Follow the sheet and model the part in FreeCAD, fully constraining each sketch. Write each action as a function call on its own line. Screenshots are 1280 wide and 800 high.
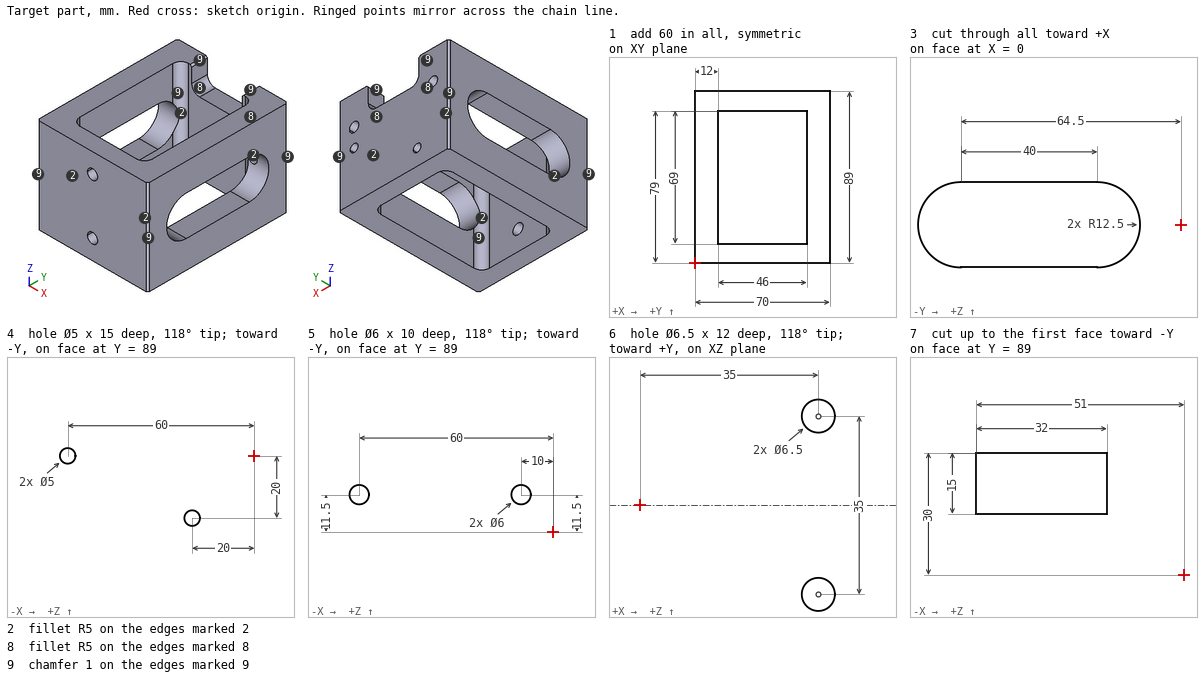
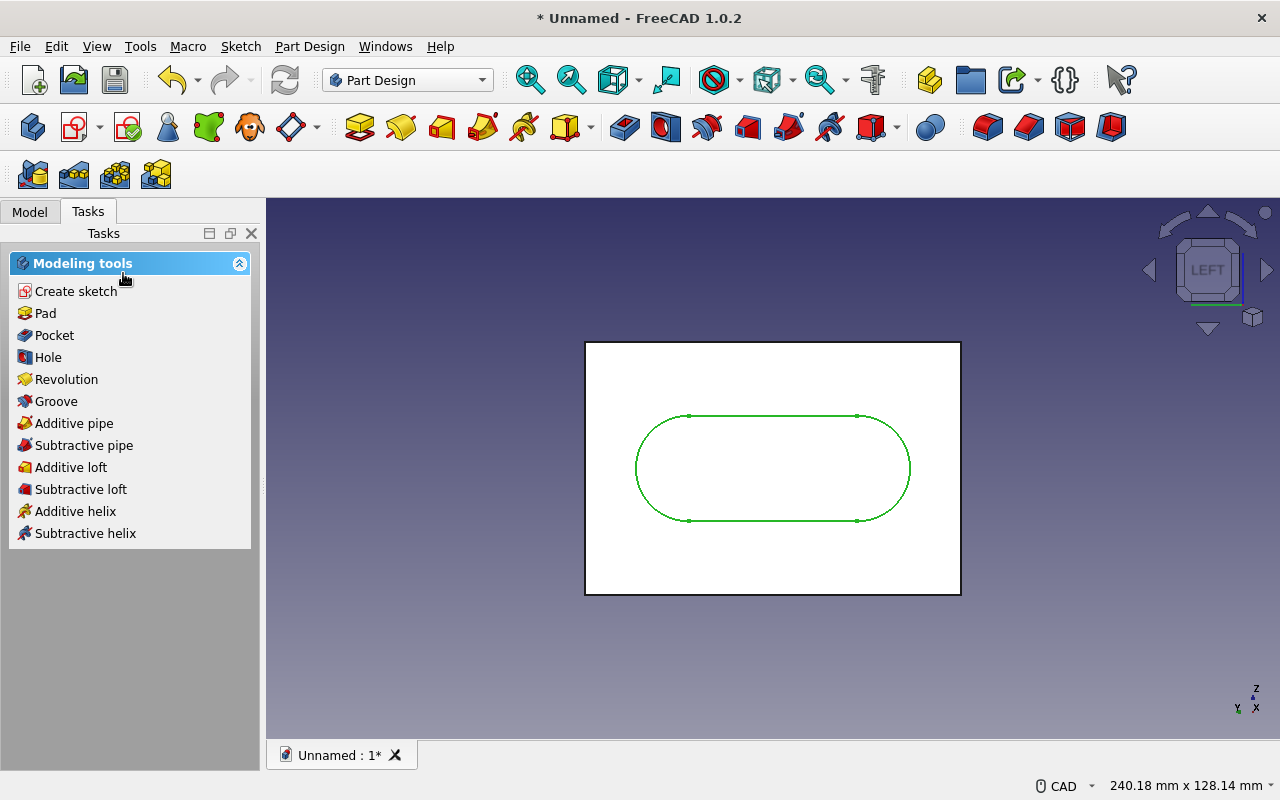
click(625, 128)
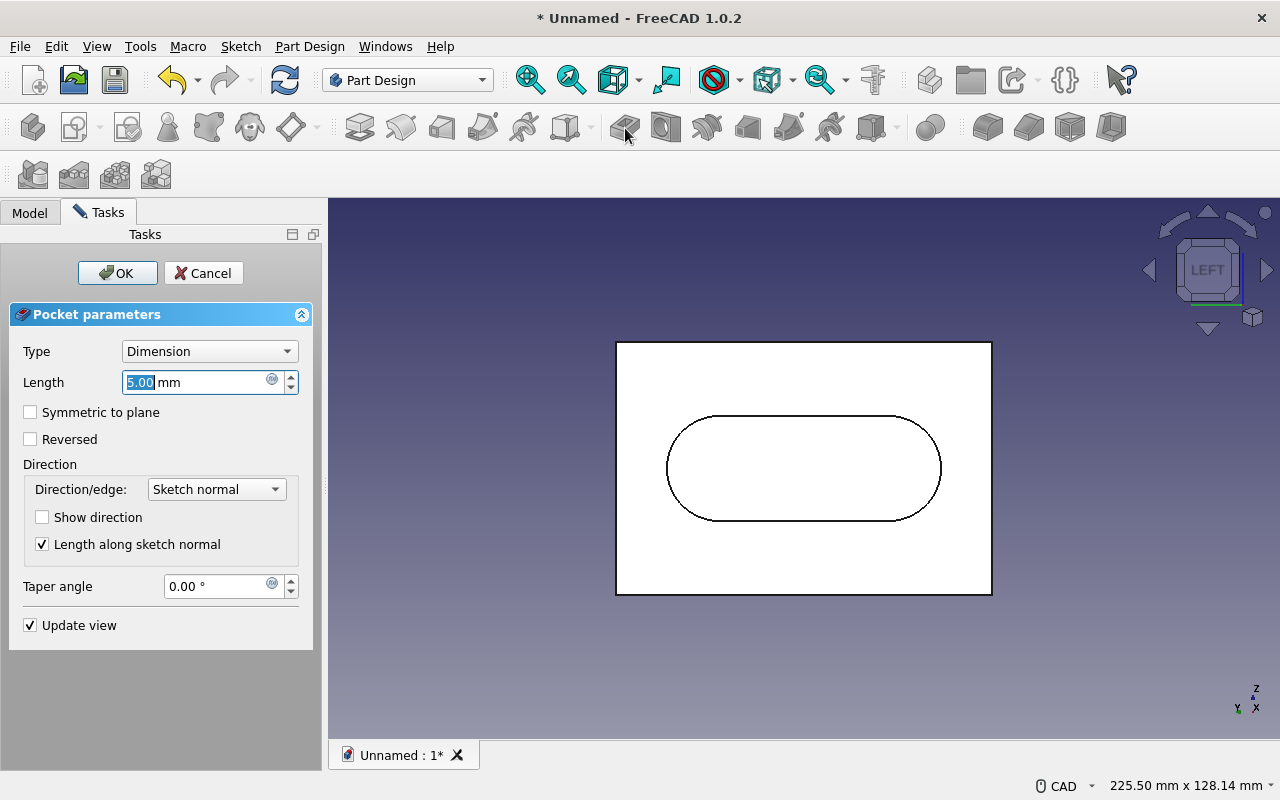
click(210, 352)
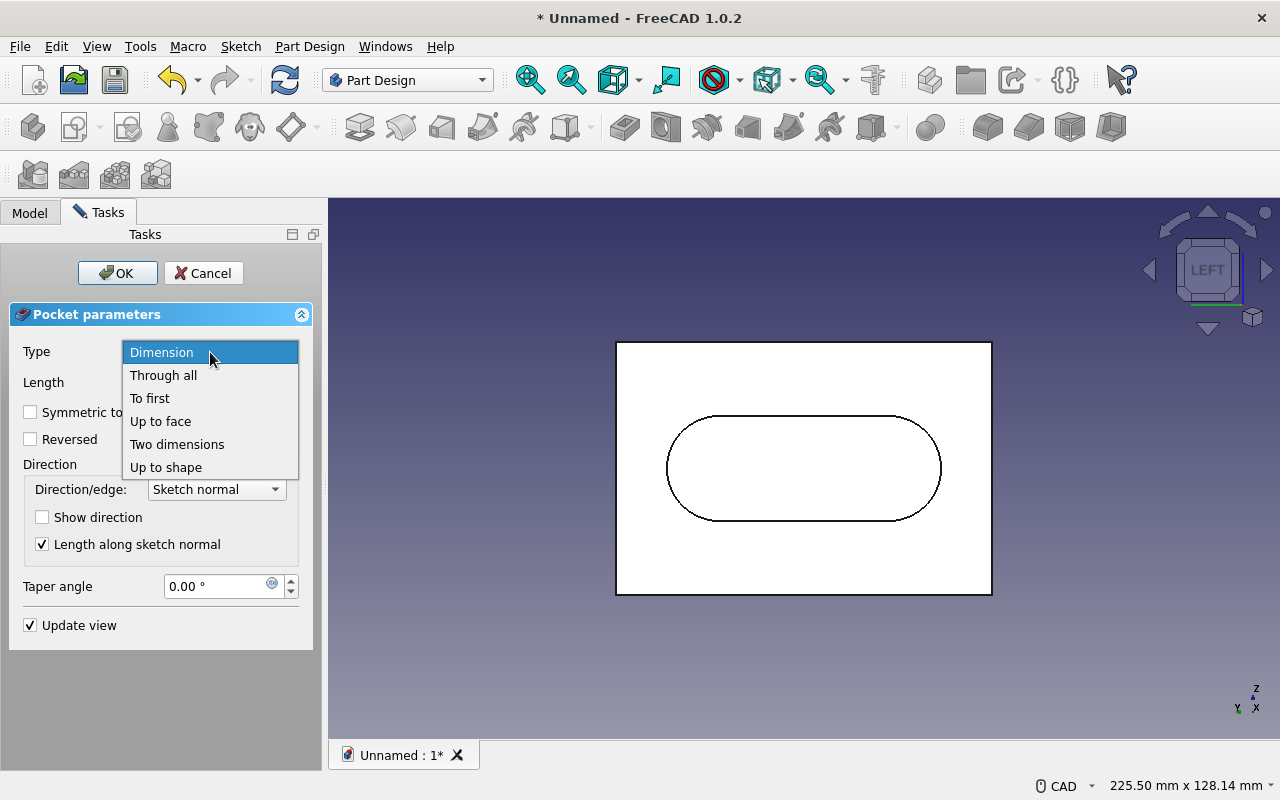
click(208, 376)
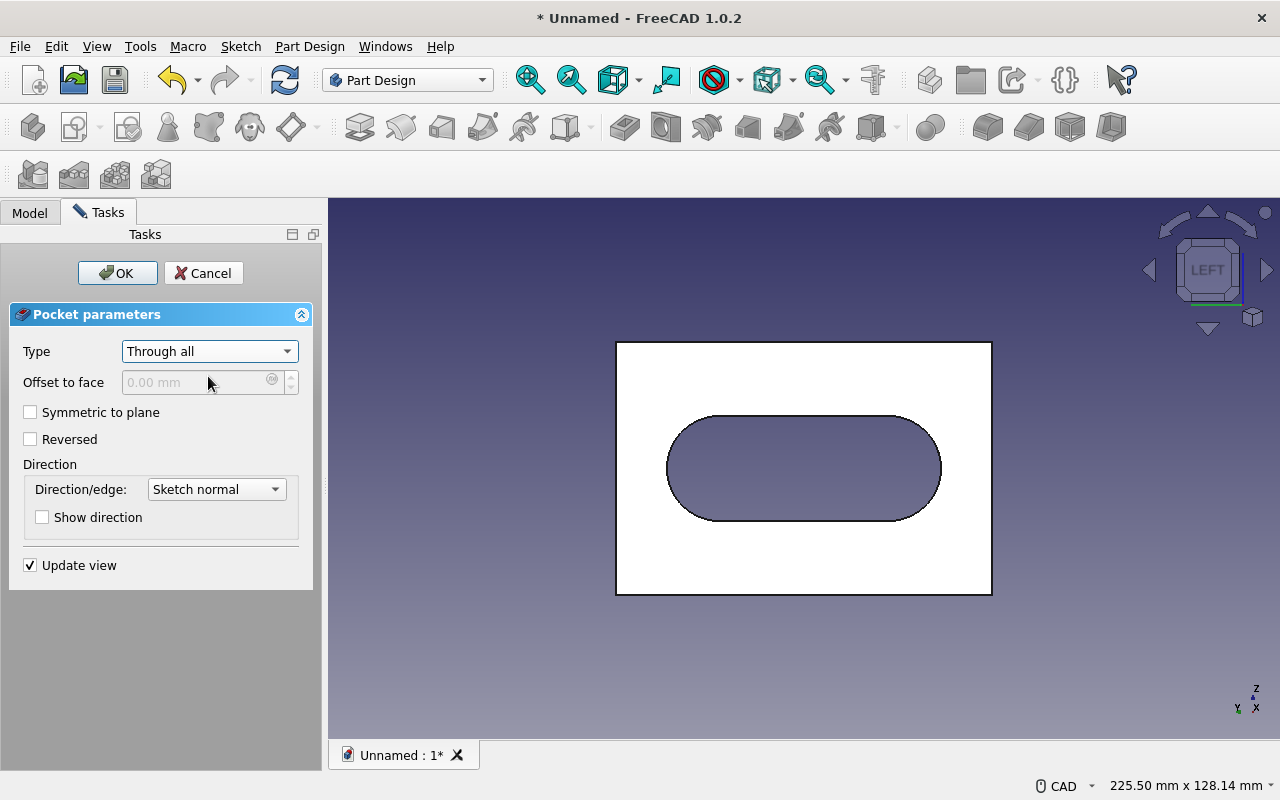
click(118, 273)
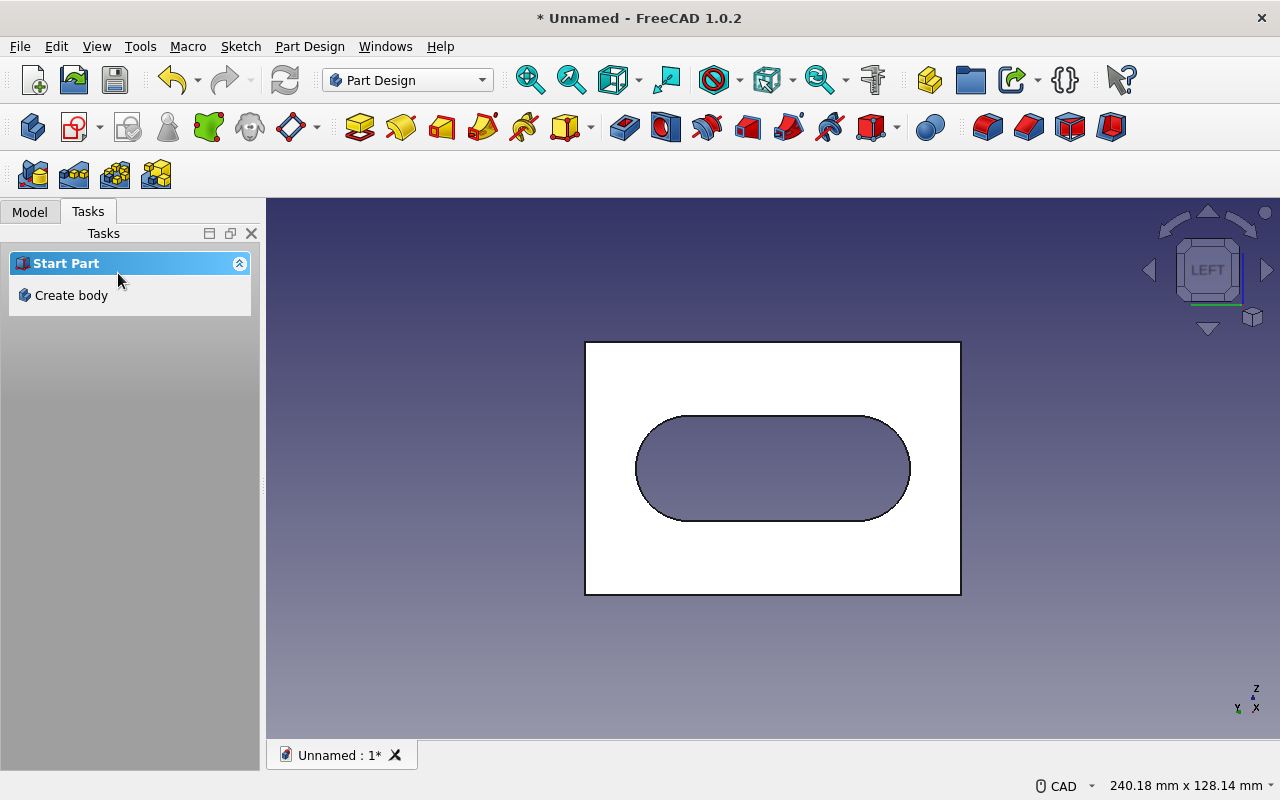
key(4)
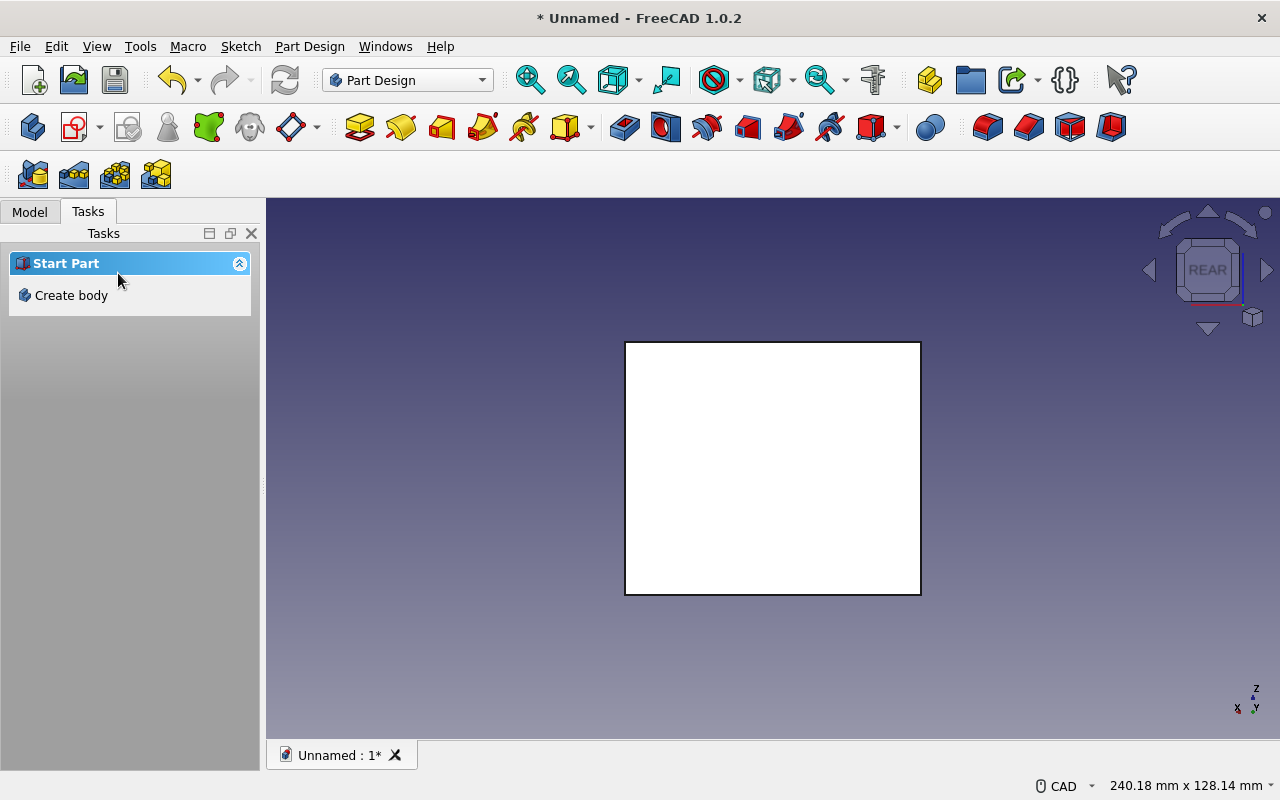
click(773, 468)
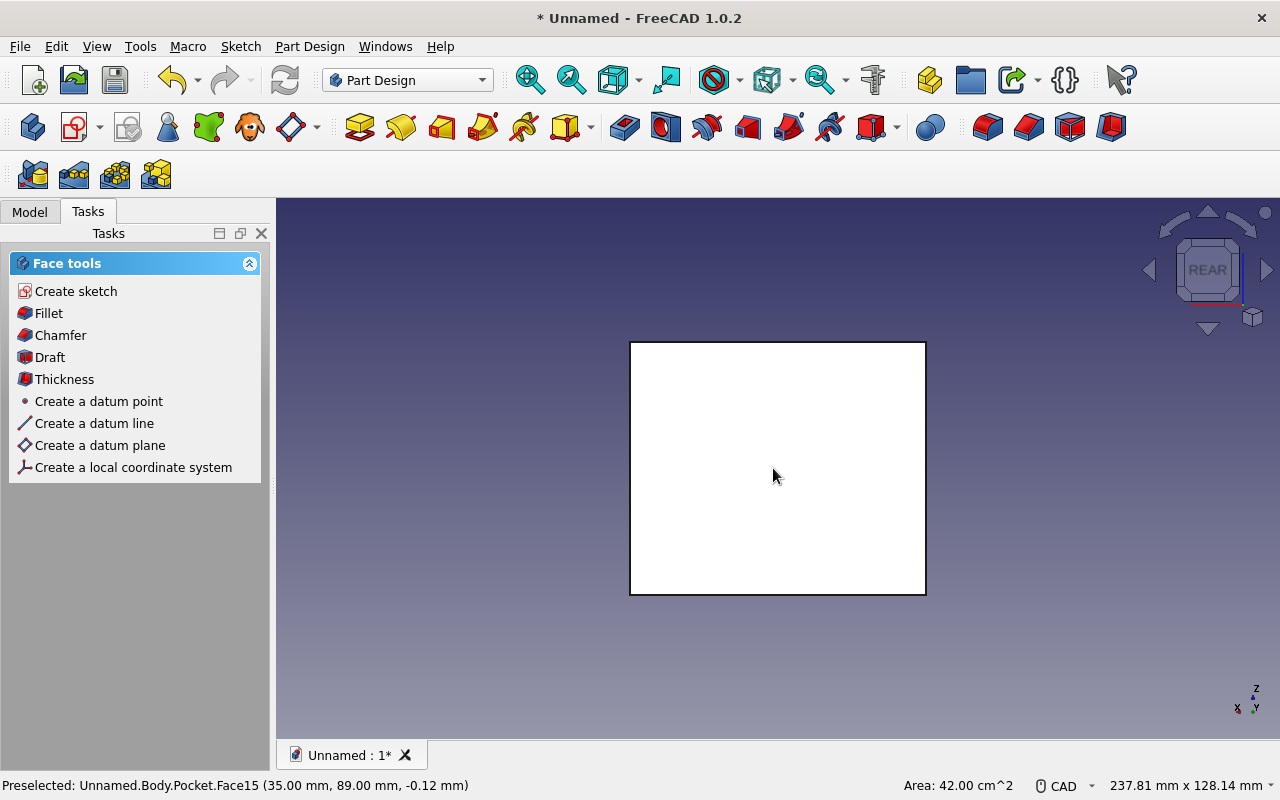
click(74, 128)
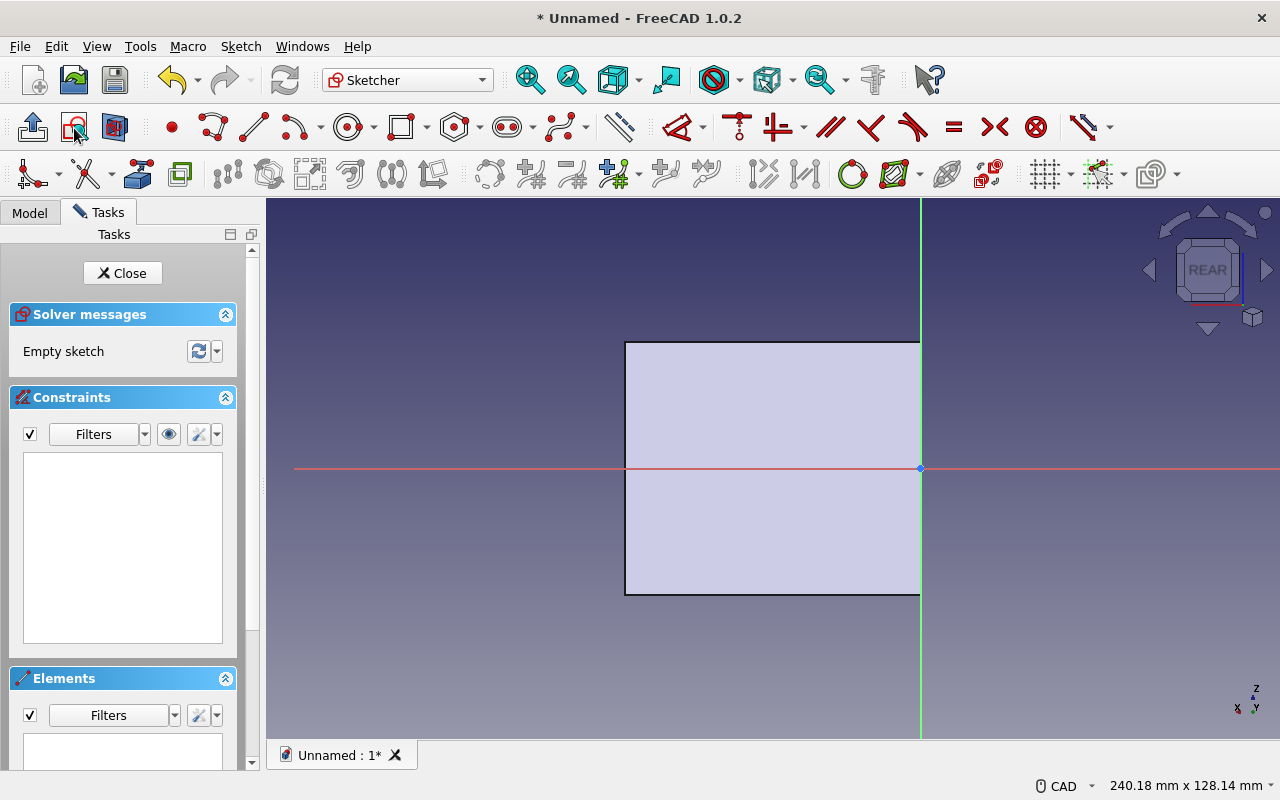
scroll(858, 545, up, 4)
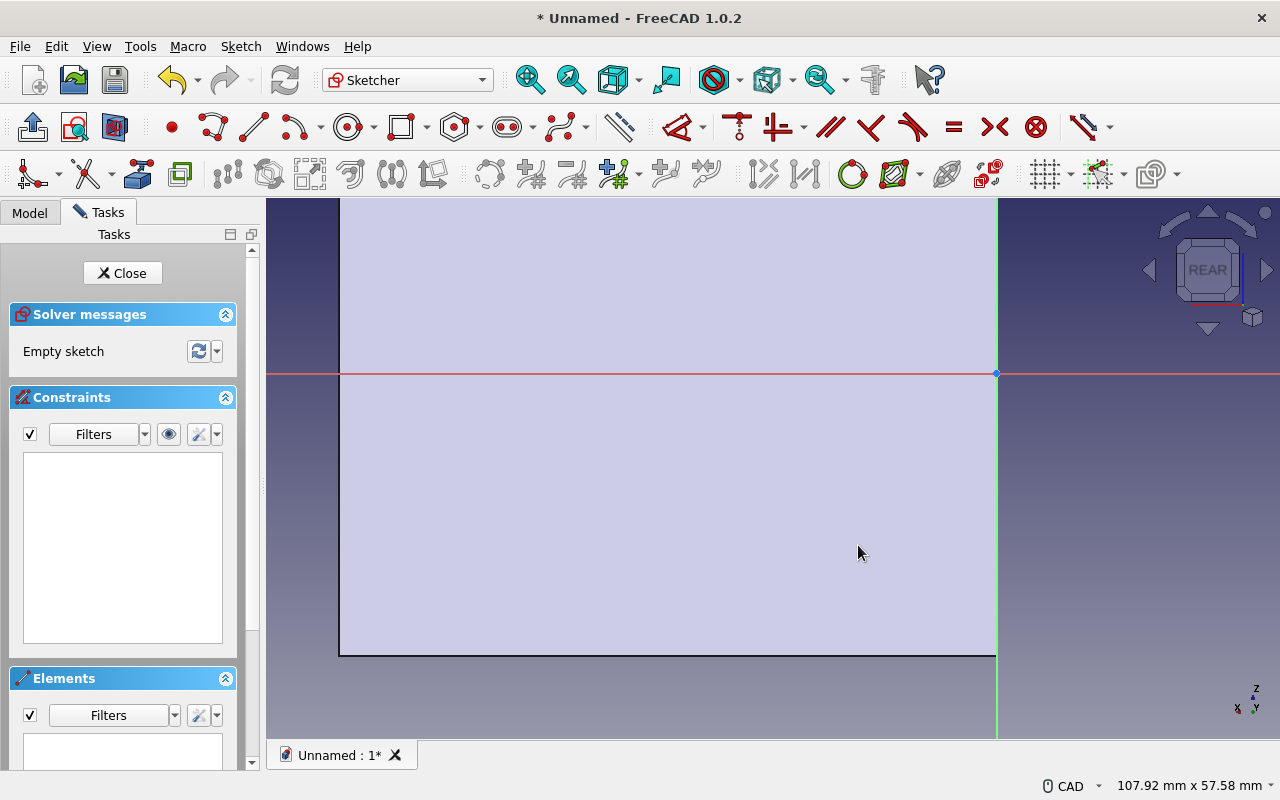
click(348, 128)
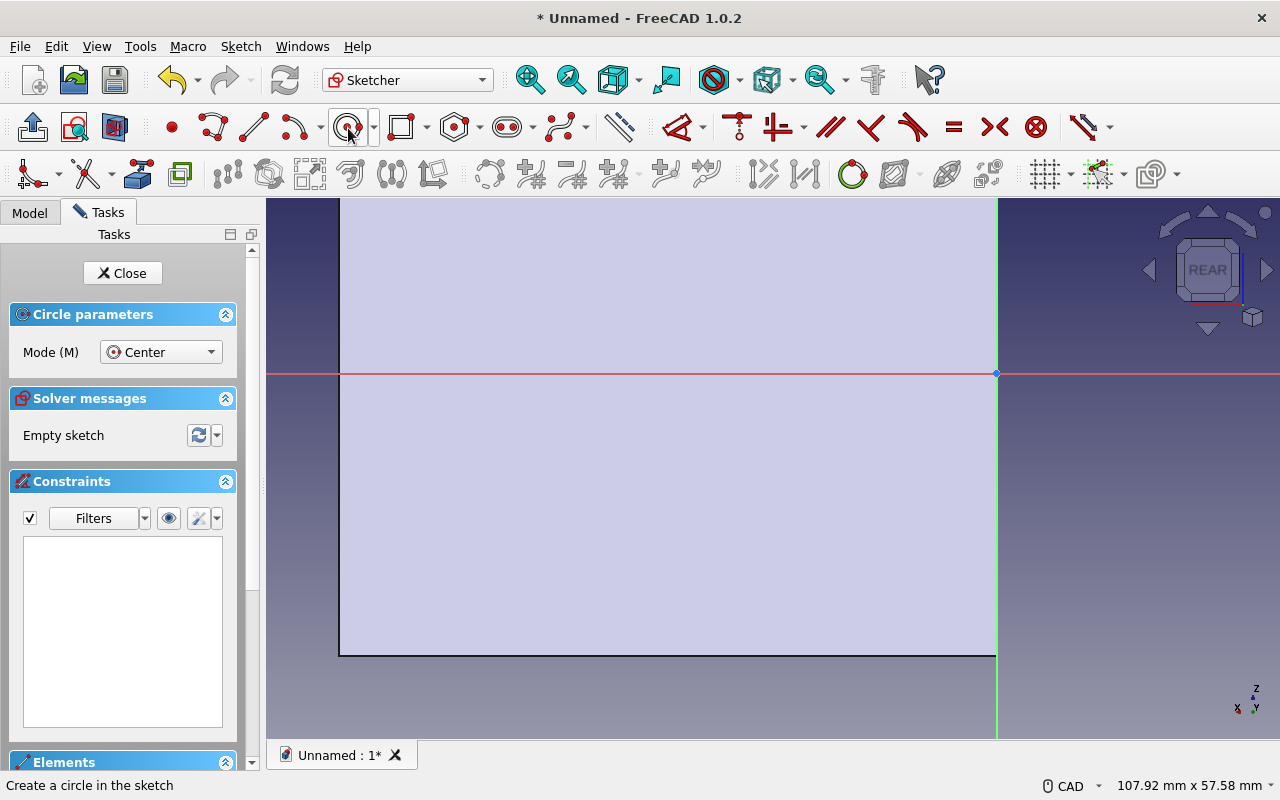
click(433, 374)
click(450, 357)